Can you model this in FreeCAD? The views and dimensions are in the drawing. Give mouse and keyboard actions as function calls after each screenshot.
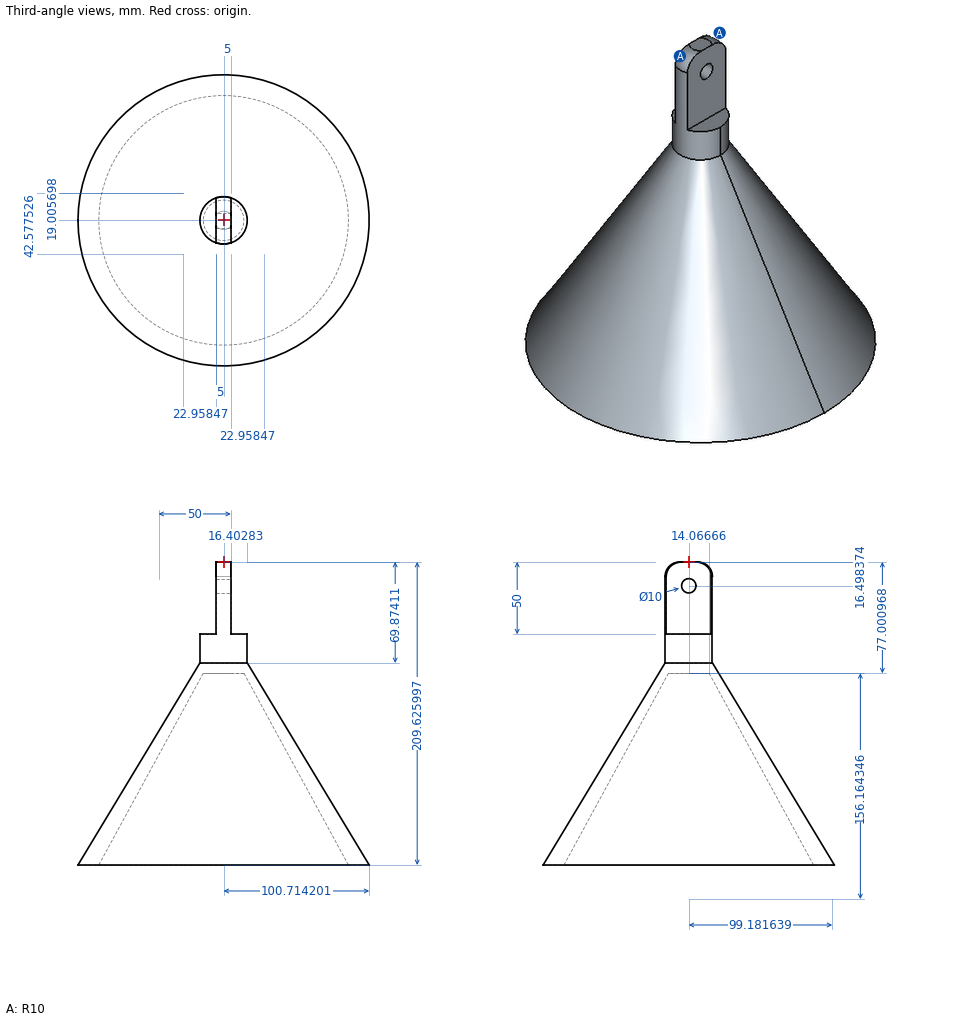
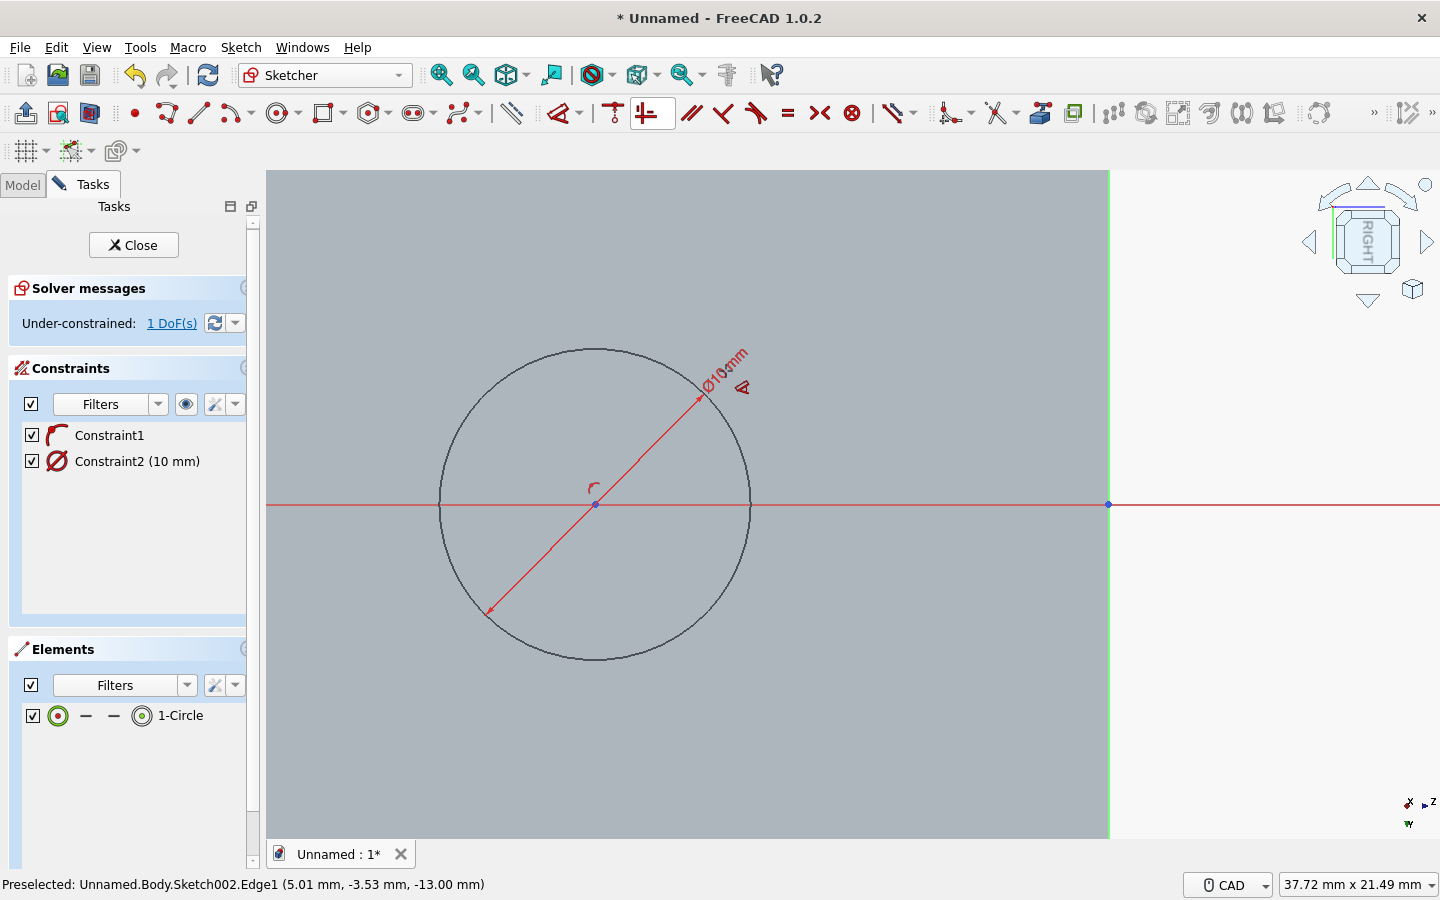
click(595, 504)
click(852, 538)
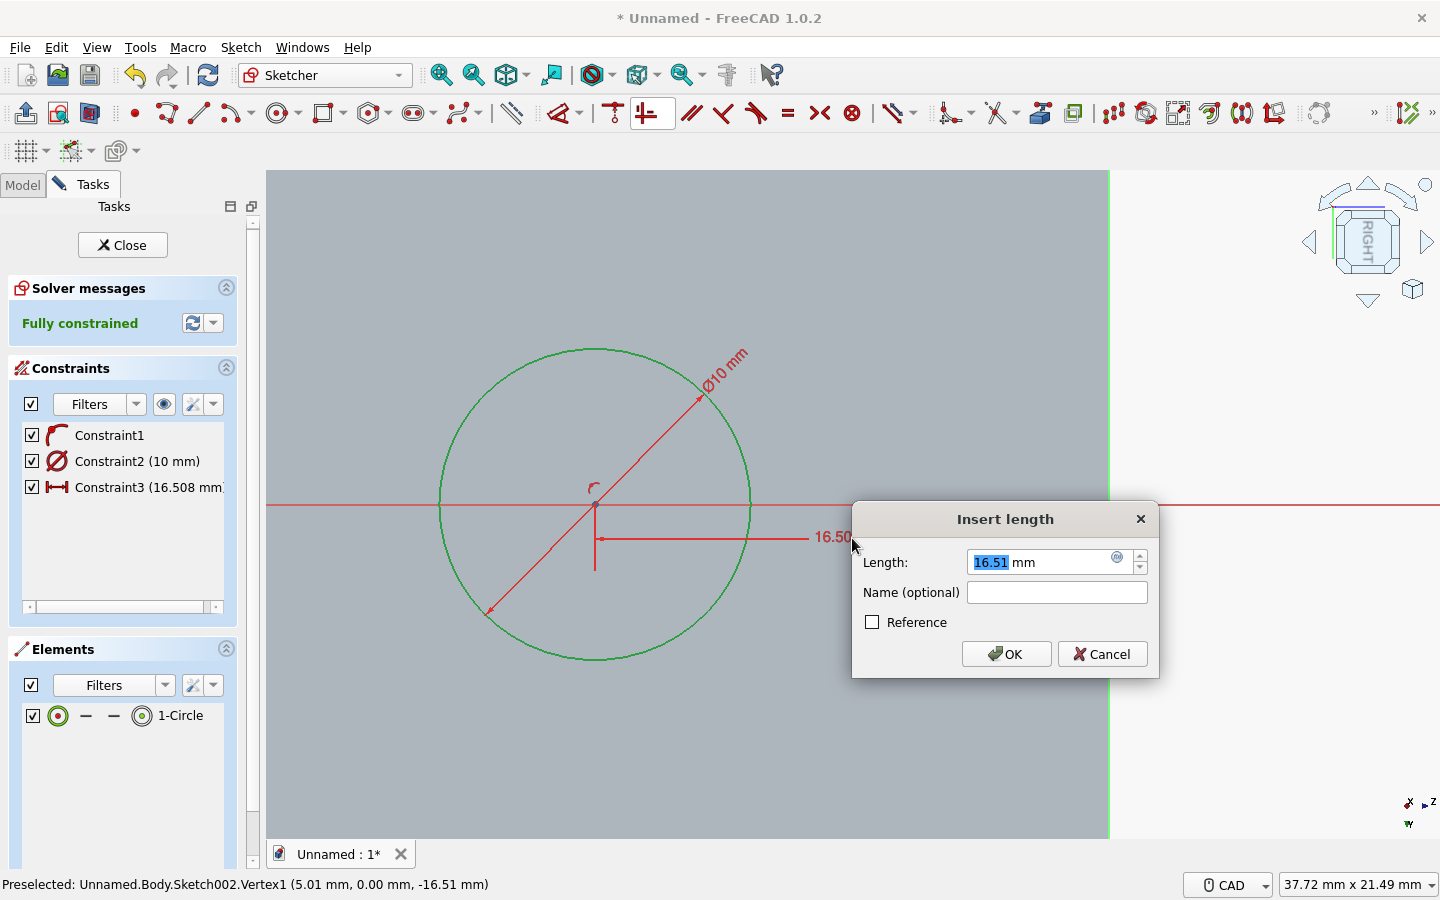
text(16.498374)
key(Return)
key(Escape)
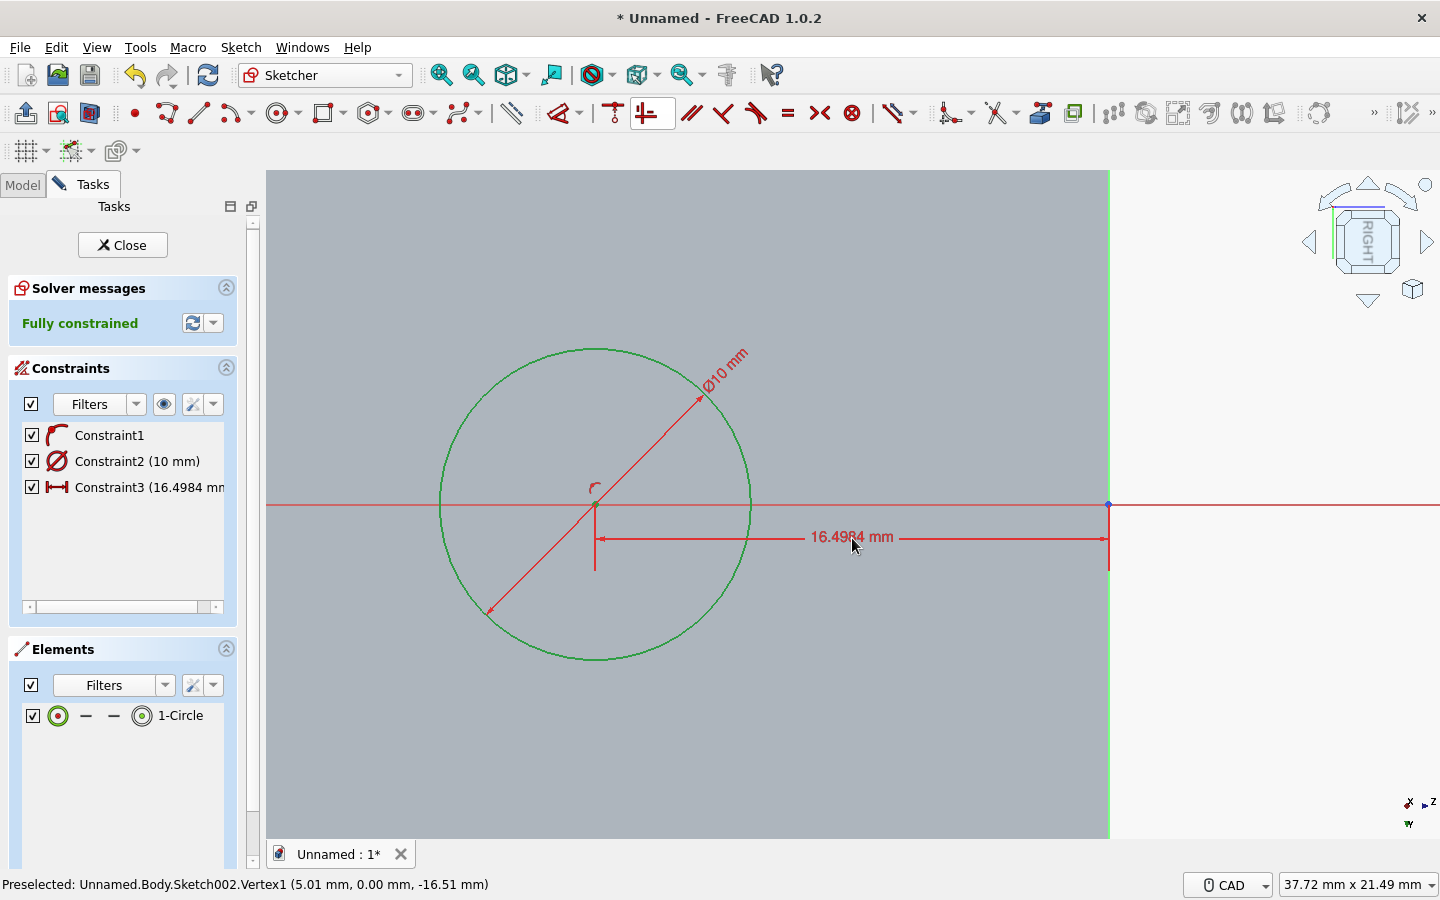
click(123, 245)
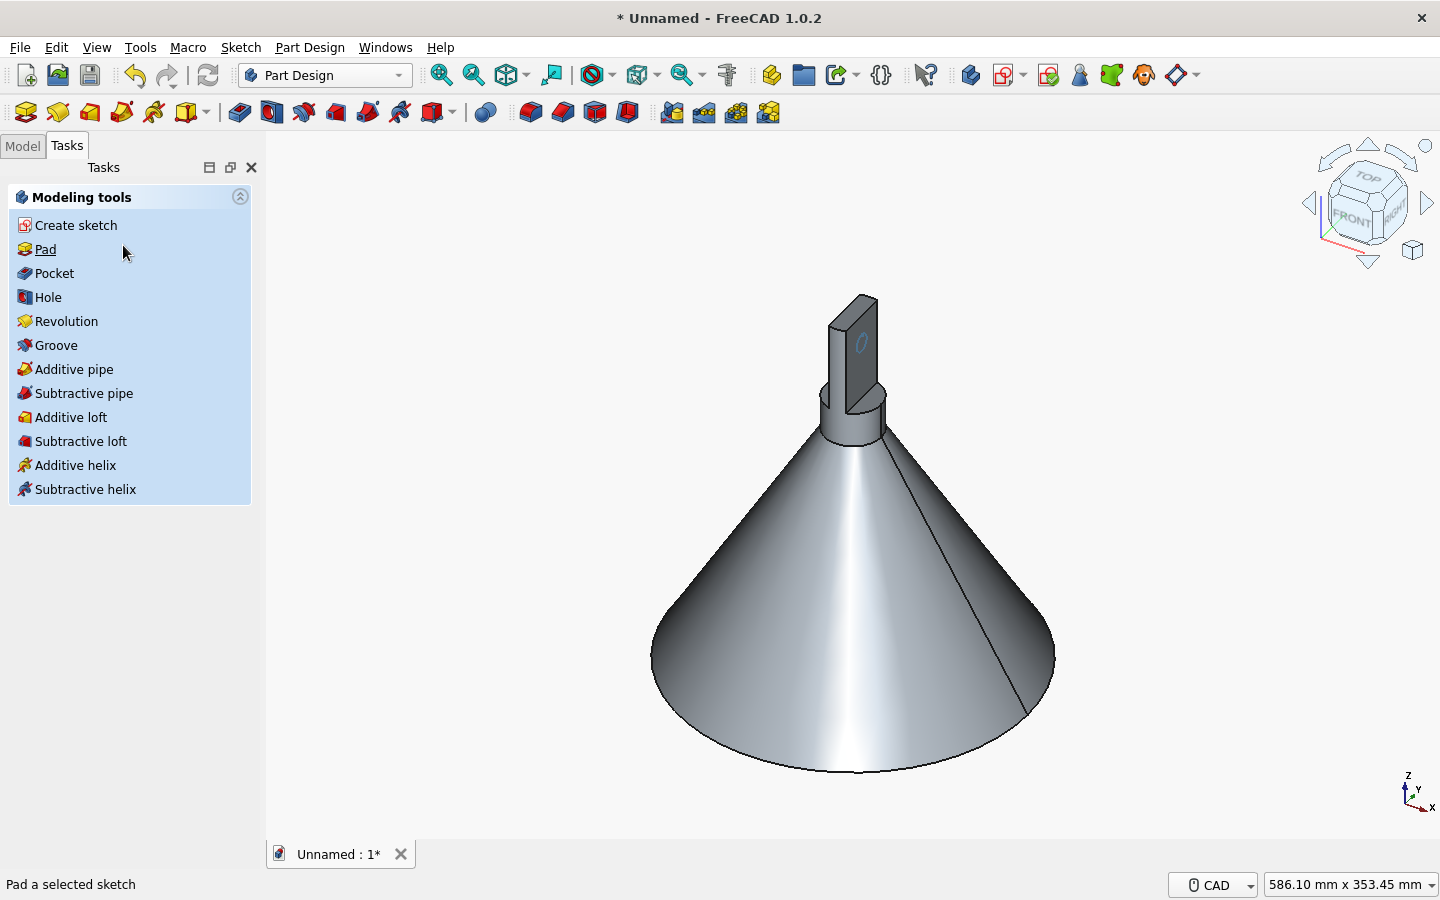
click(240, 112)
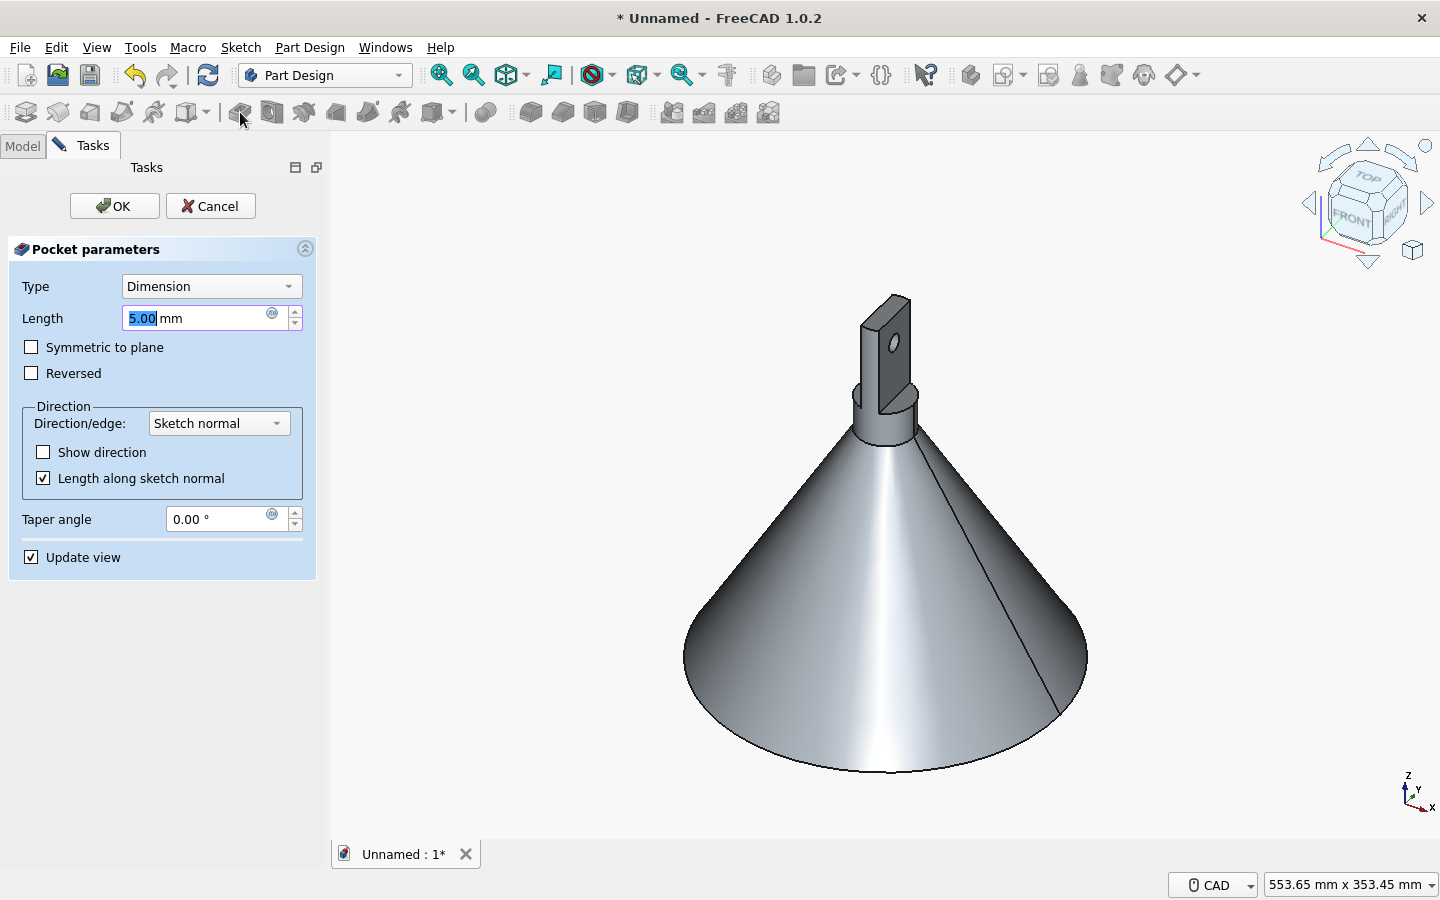
text(50)
key(Tab)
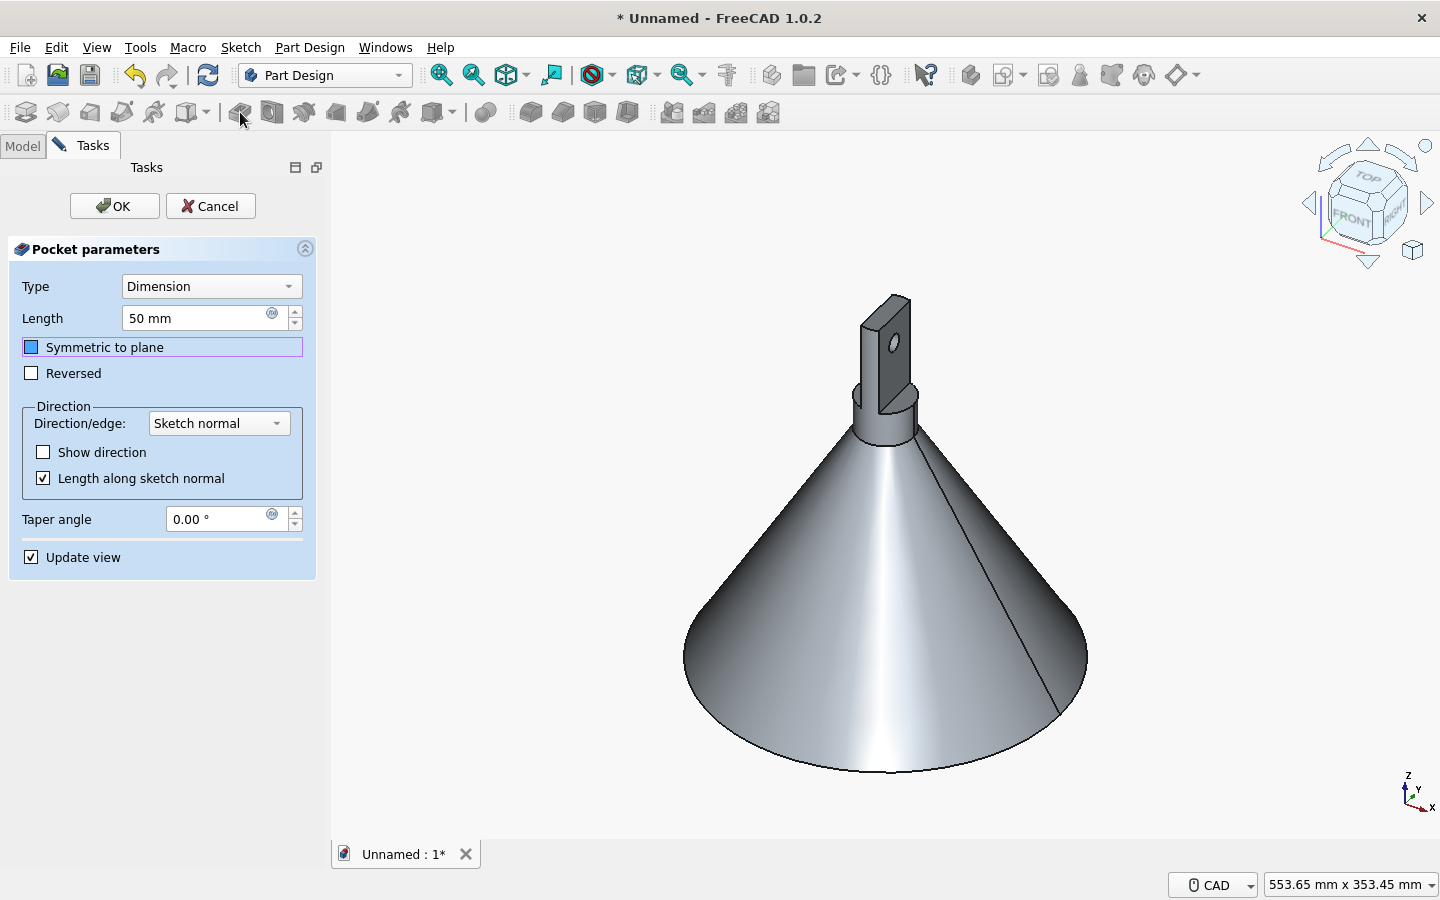
click(115, 206)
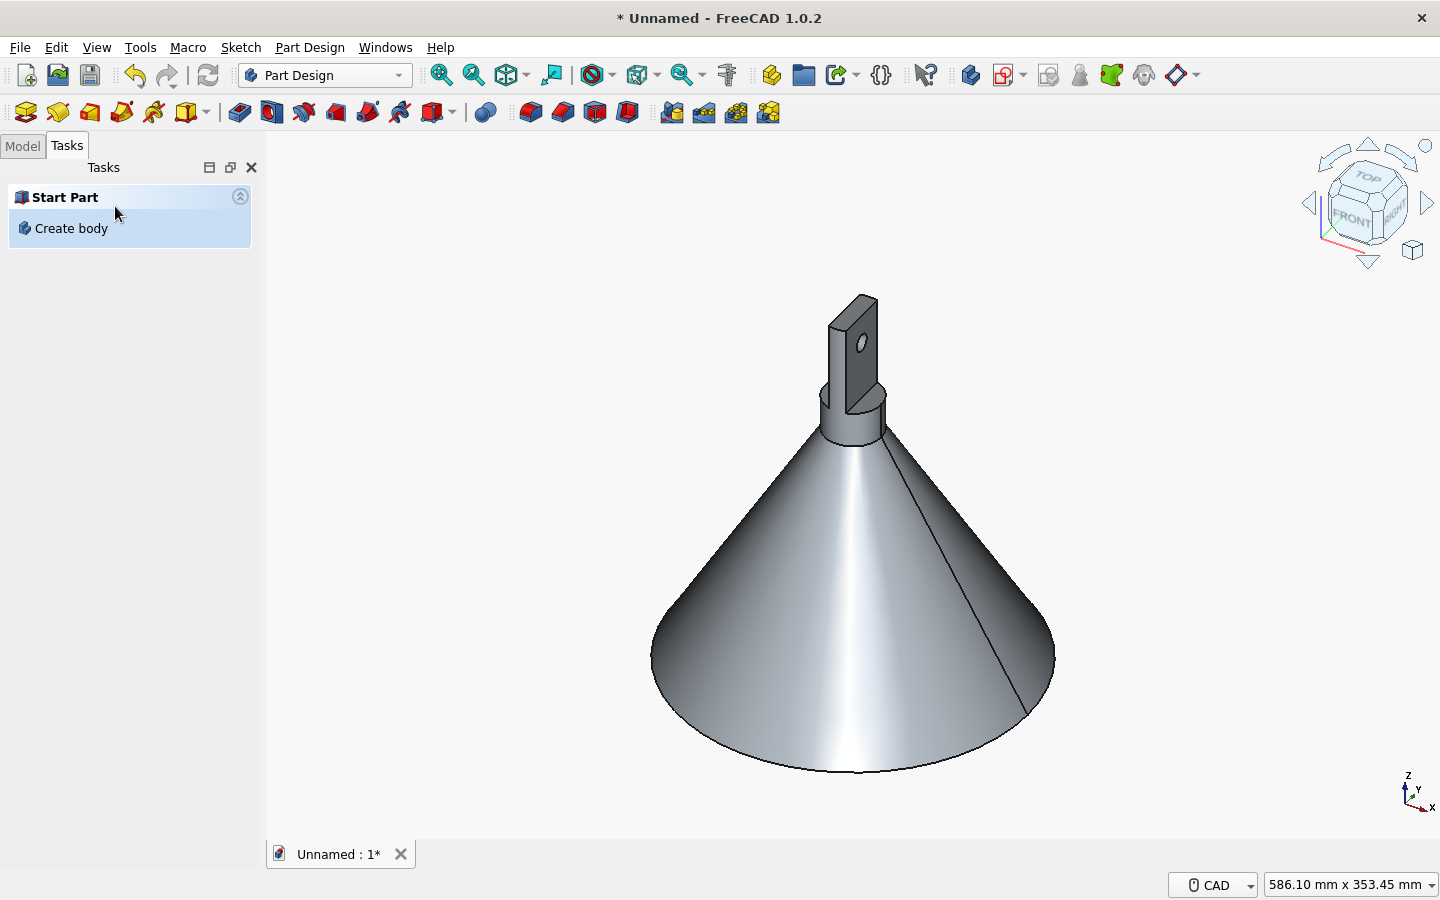
click(837, 328)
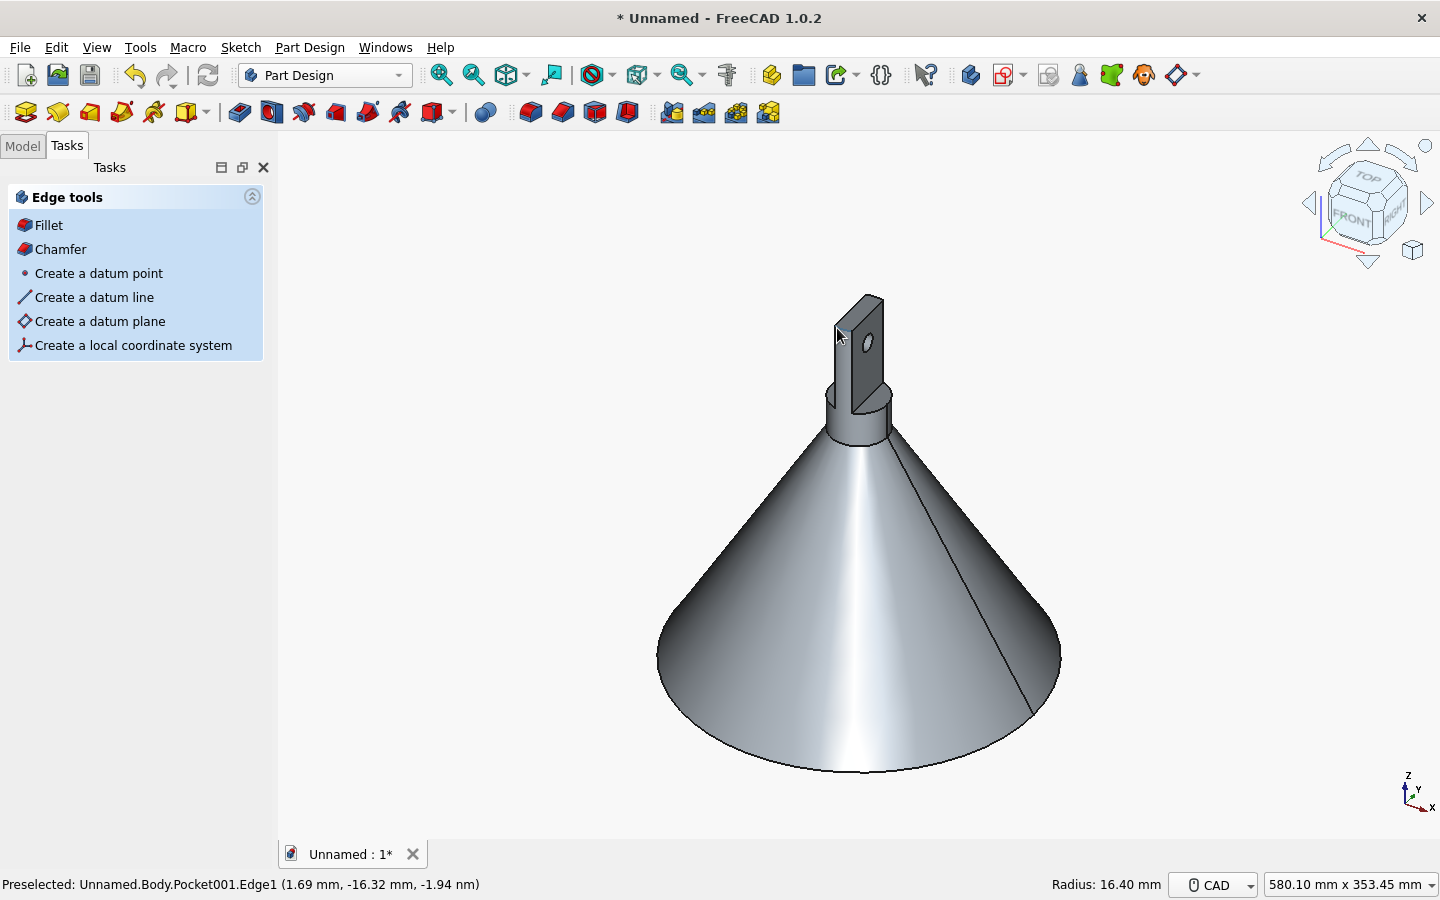
scroll(875, 296, up, 4)